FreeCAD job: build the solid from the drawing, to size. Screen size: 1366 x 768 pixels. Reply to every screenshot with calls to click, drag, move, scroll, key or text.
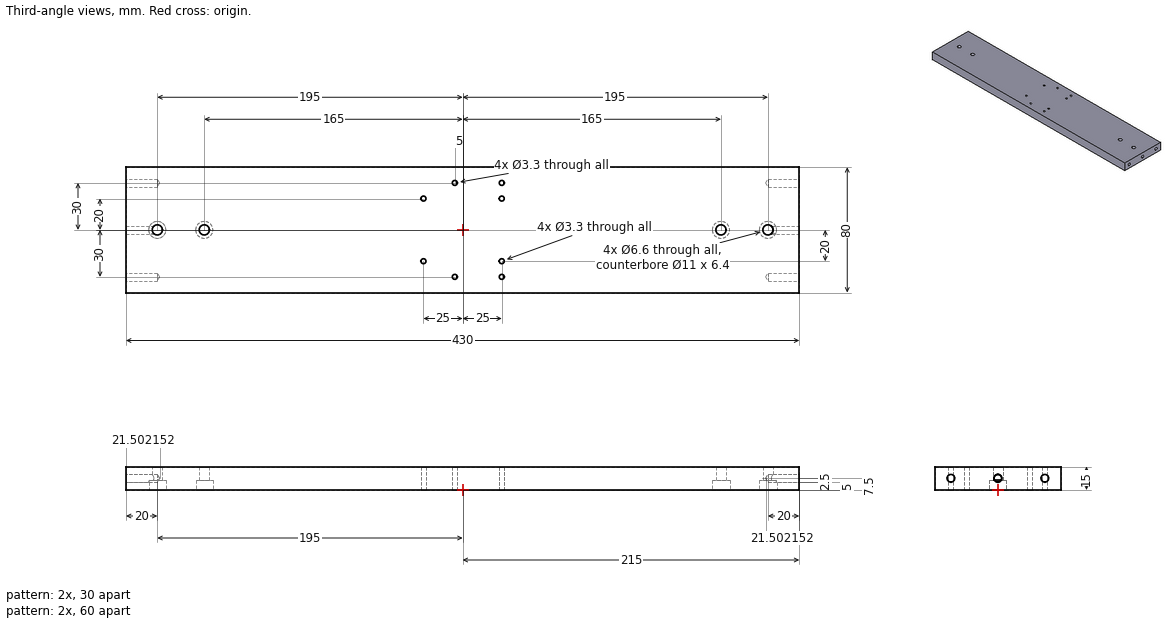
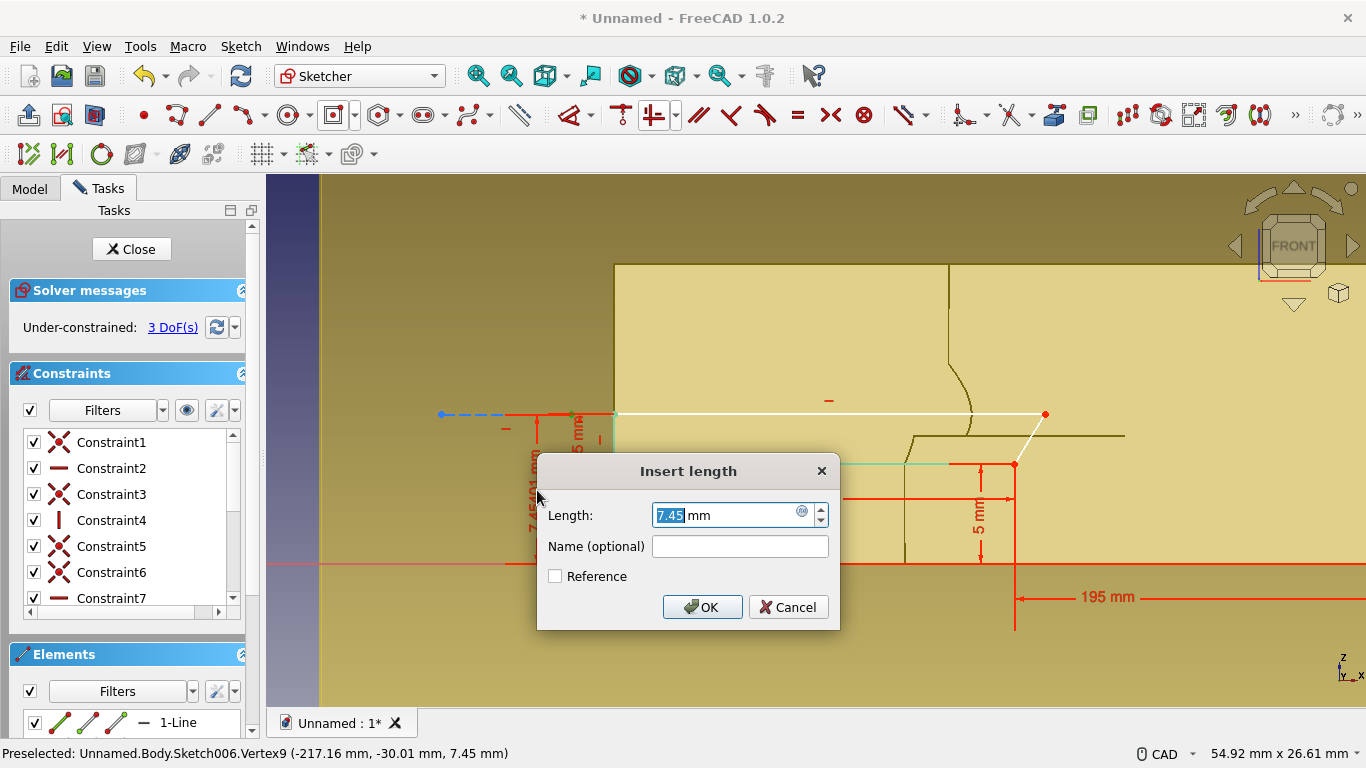
text(7.5)
key(Return)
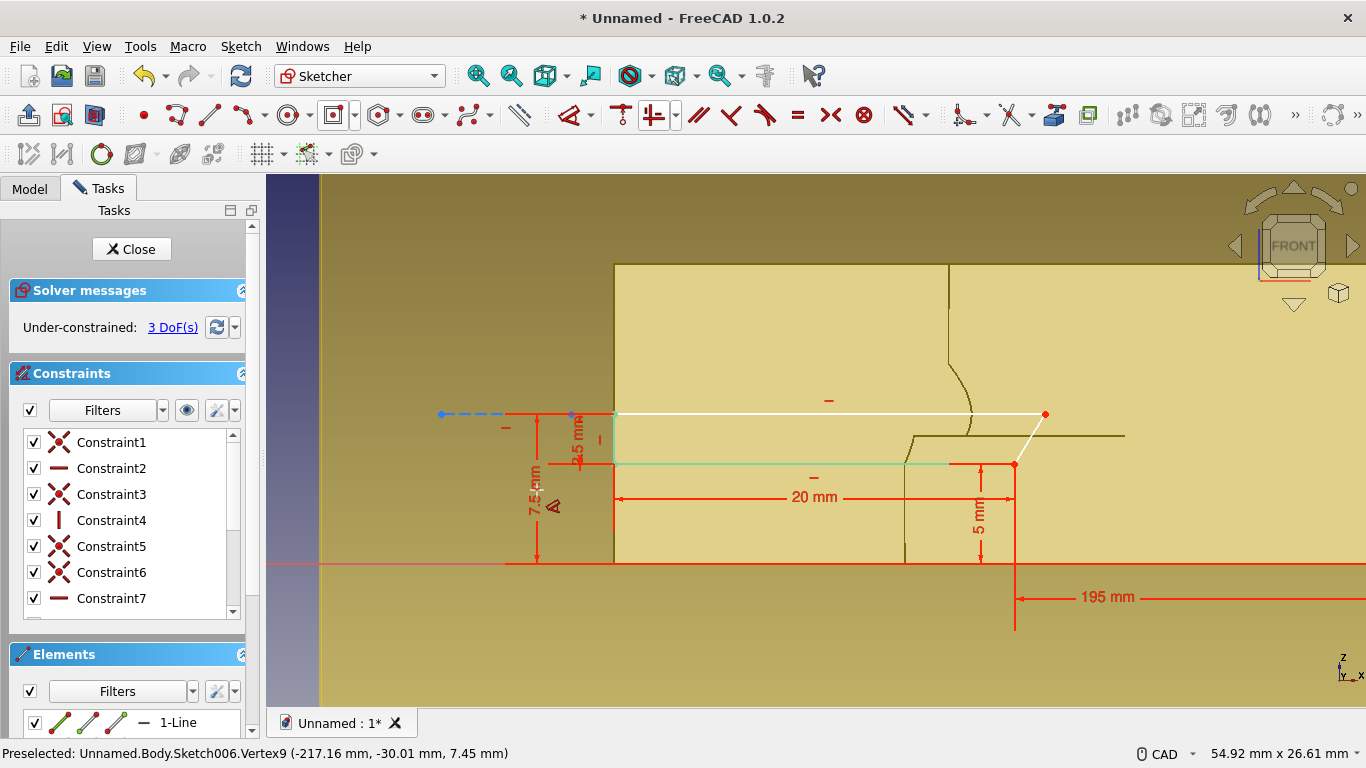
click(743, 414)
click(830, 380)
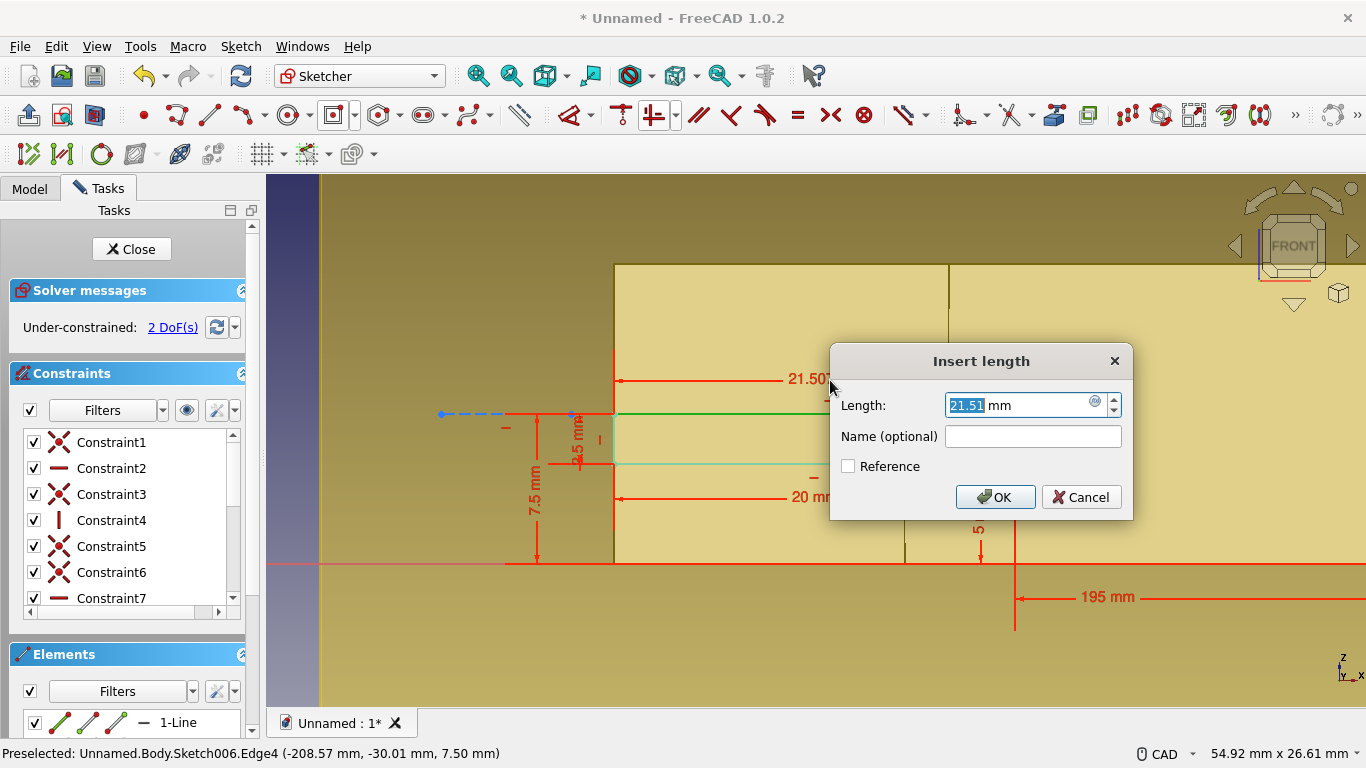
text(21.502152)
key(Return)
key(Escape)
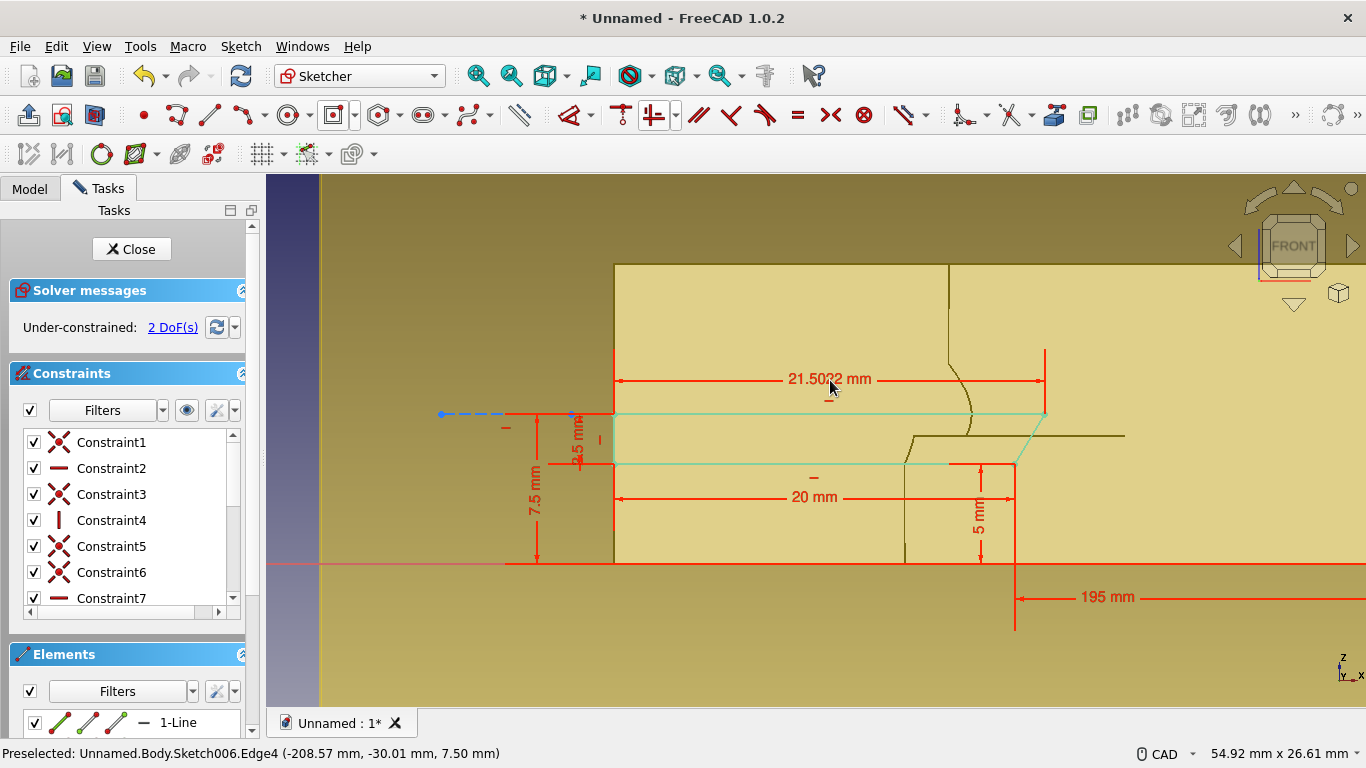
click(132, 249)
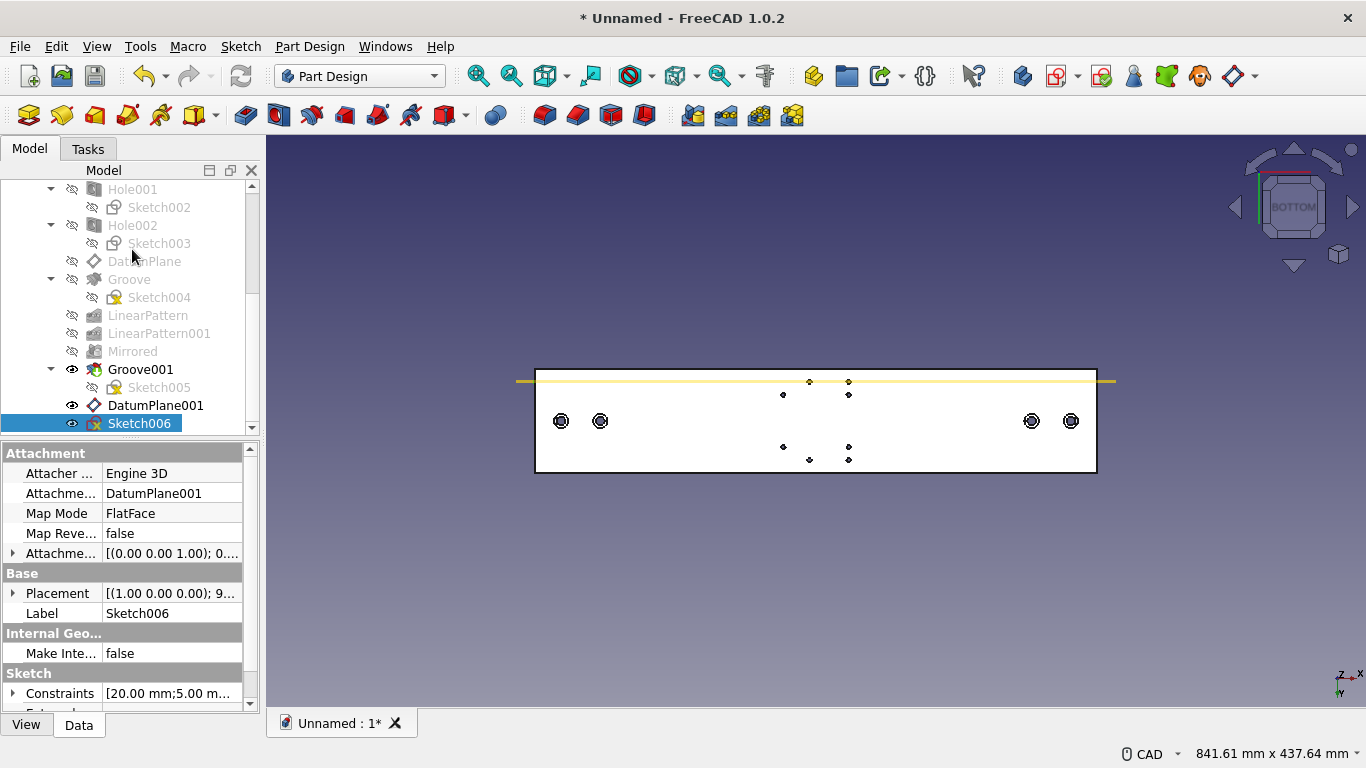
click(312, 116)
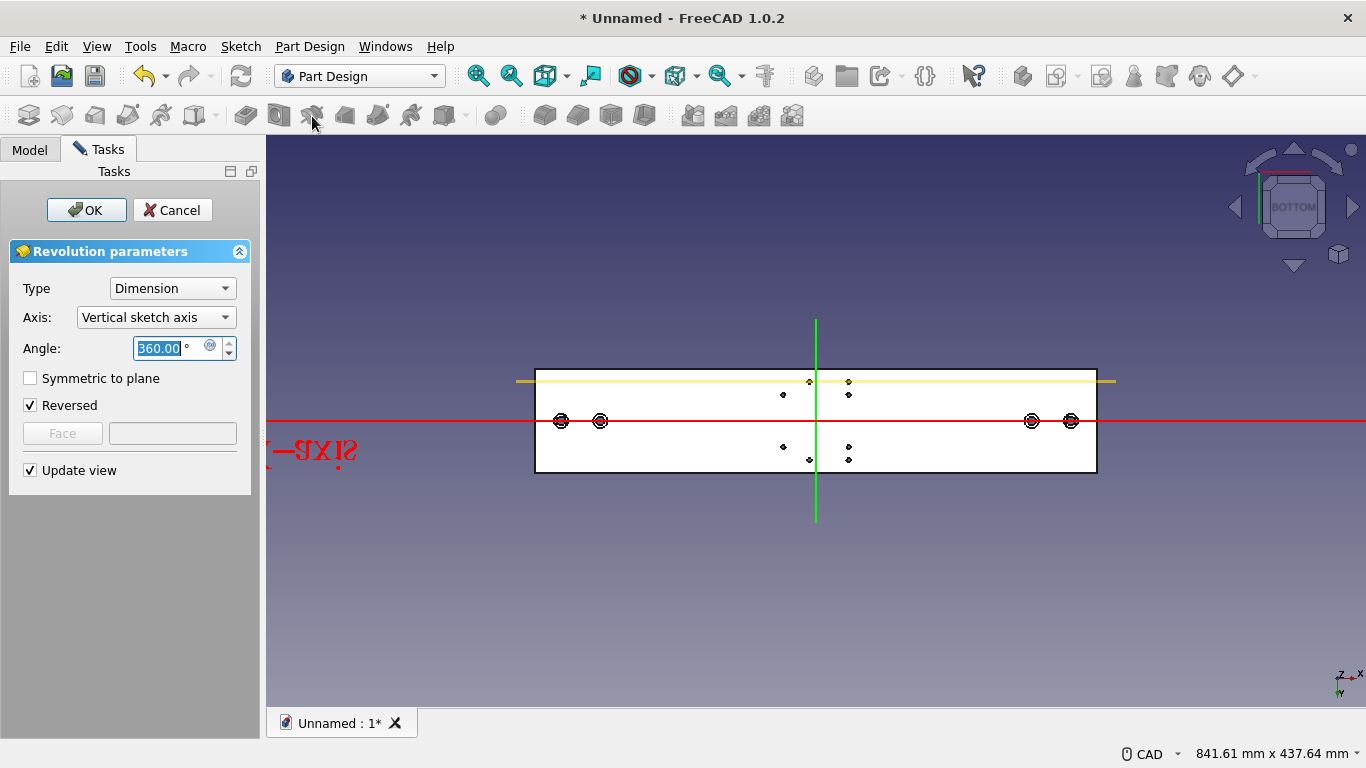
click(157, 318)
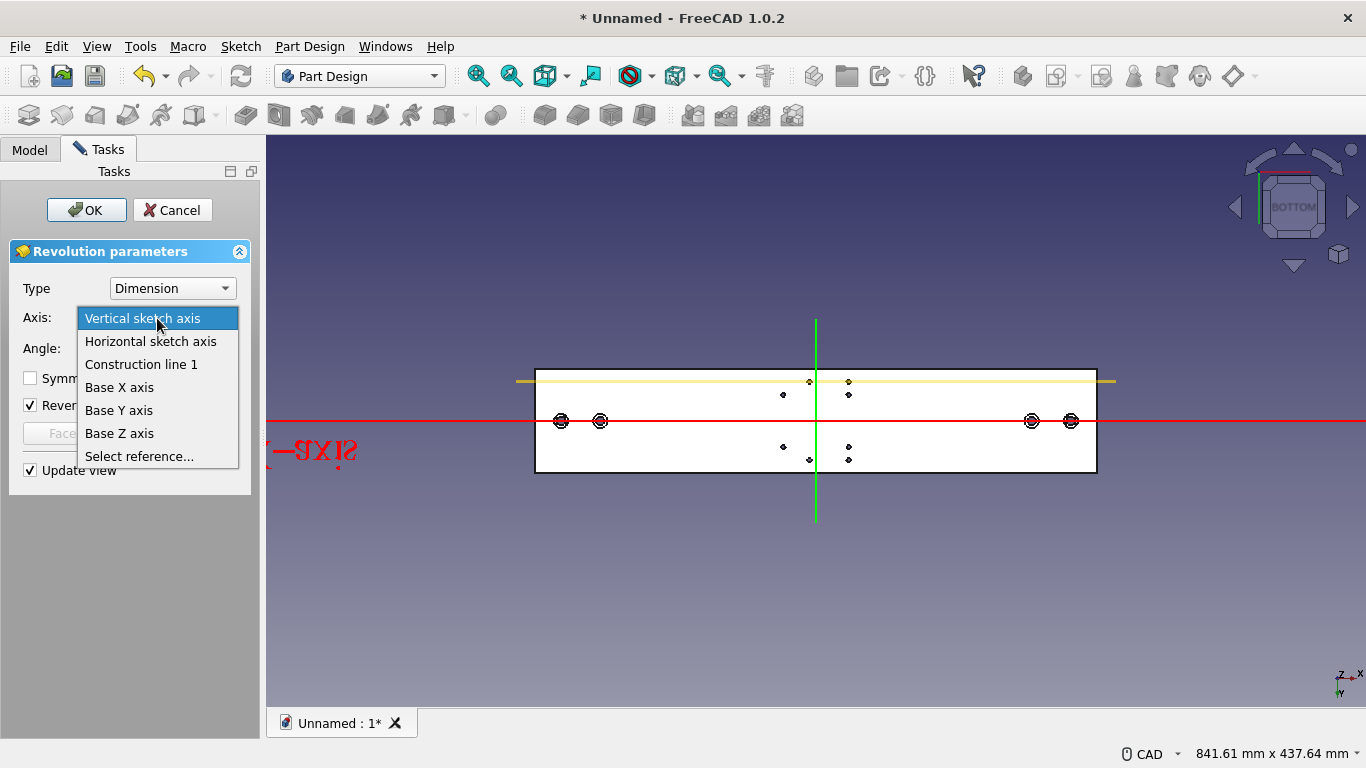
click(156, 364)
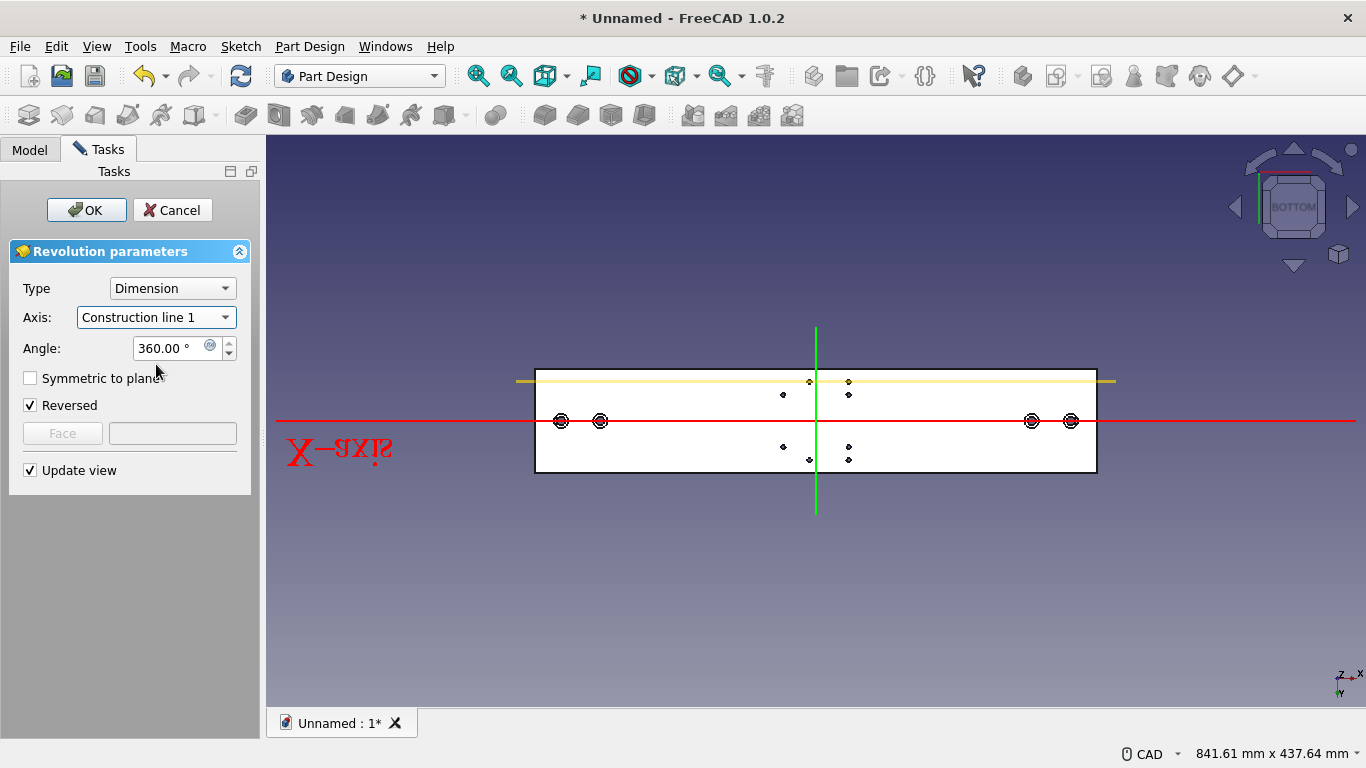
click(87, 210)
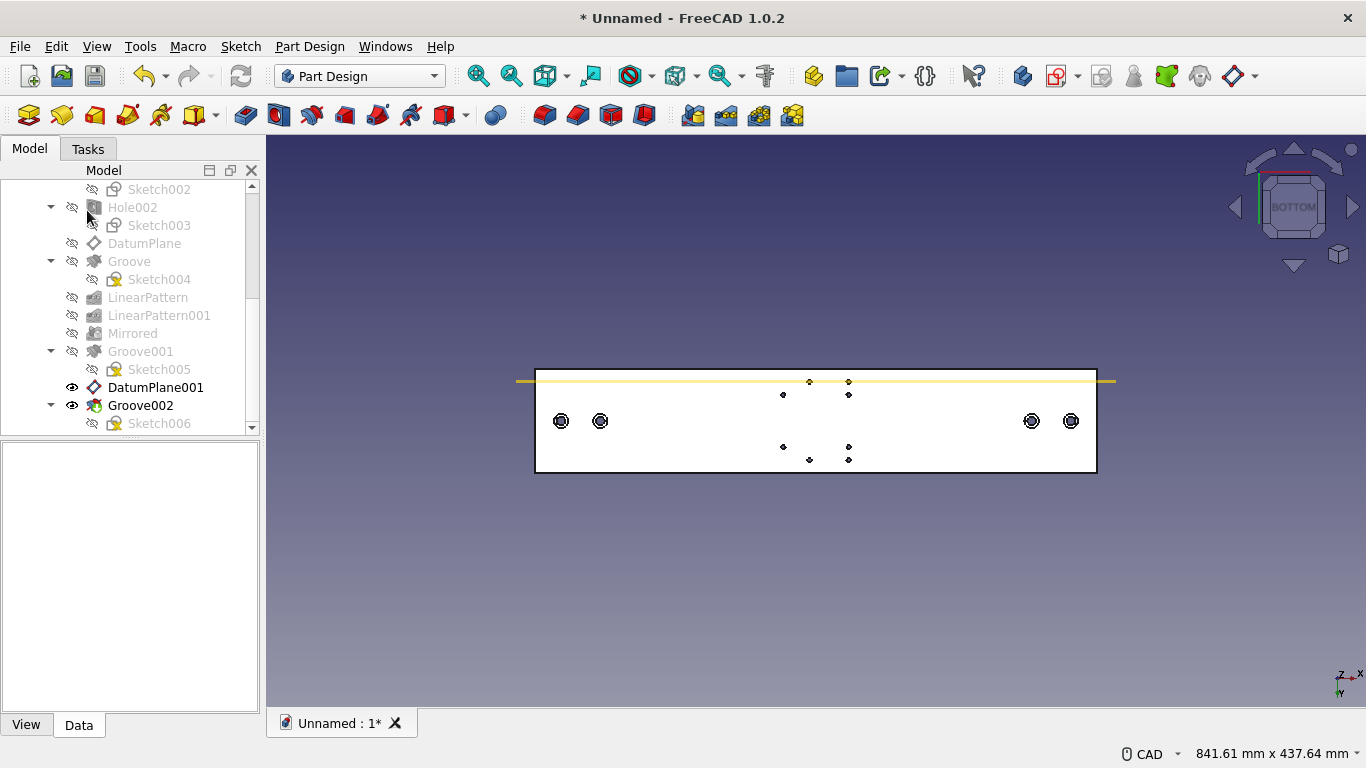
click(117, 387)
key(space)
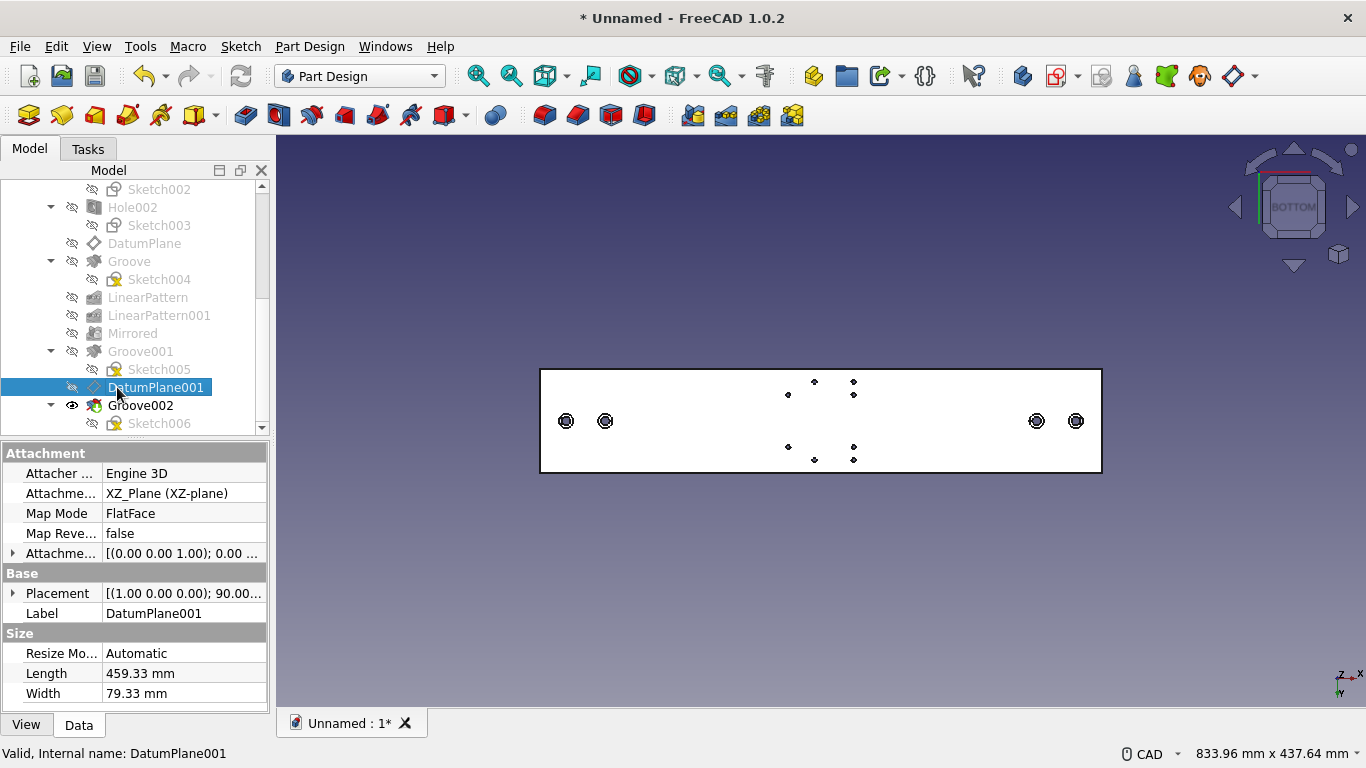
key(0)